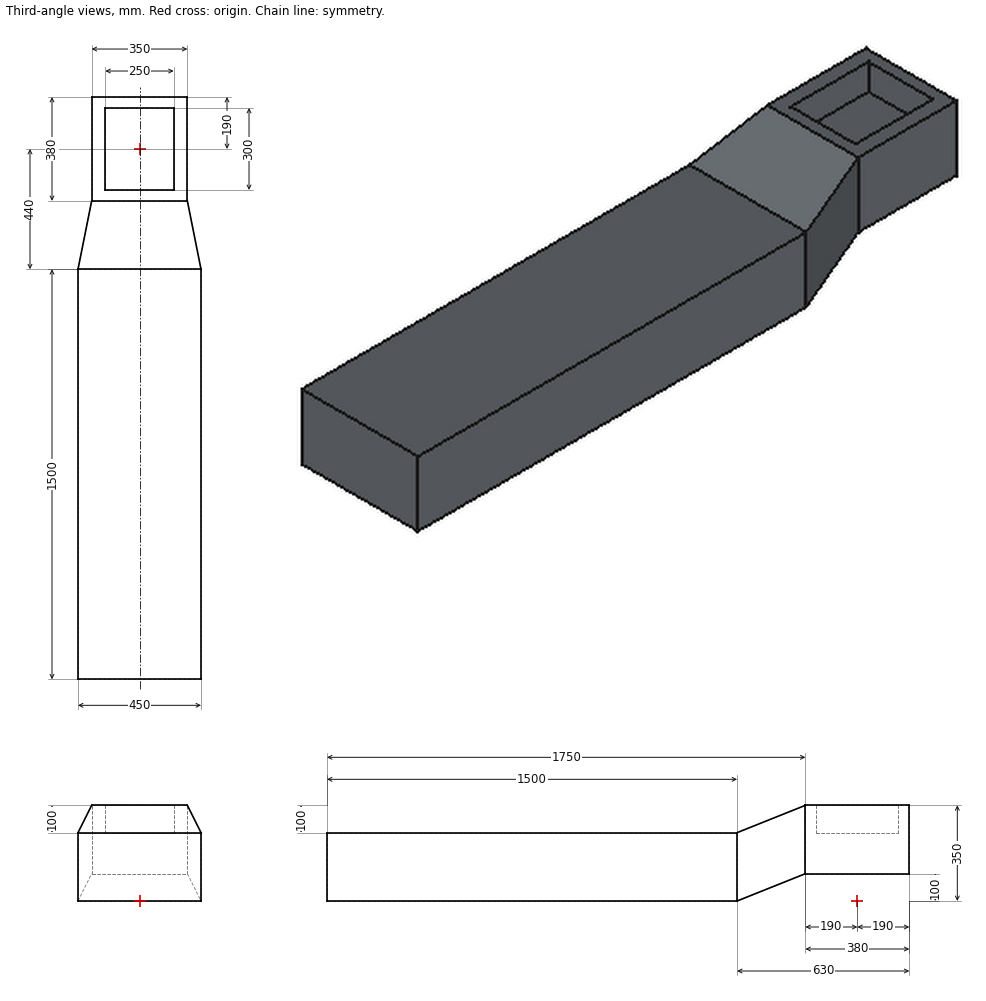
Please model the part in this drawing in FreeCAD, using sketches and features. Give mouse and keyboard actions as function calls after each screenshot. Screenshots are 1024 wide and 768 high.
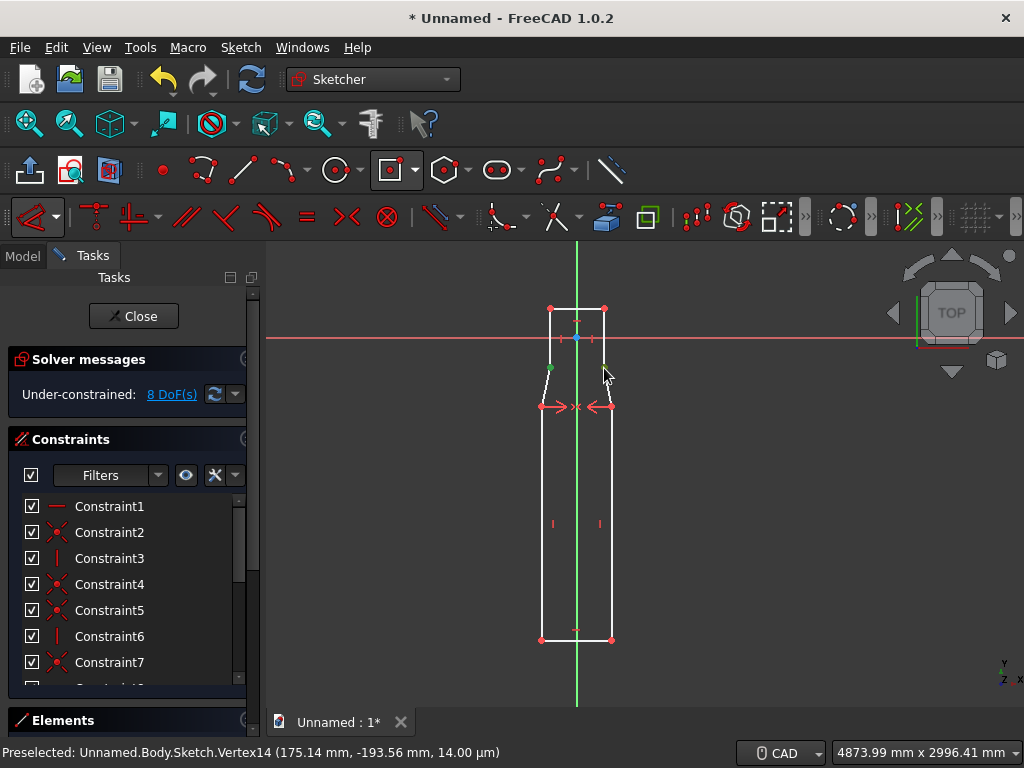
click(577, 591)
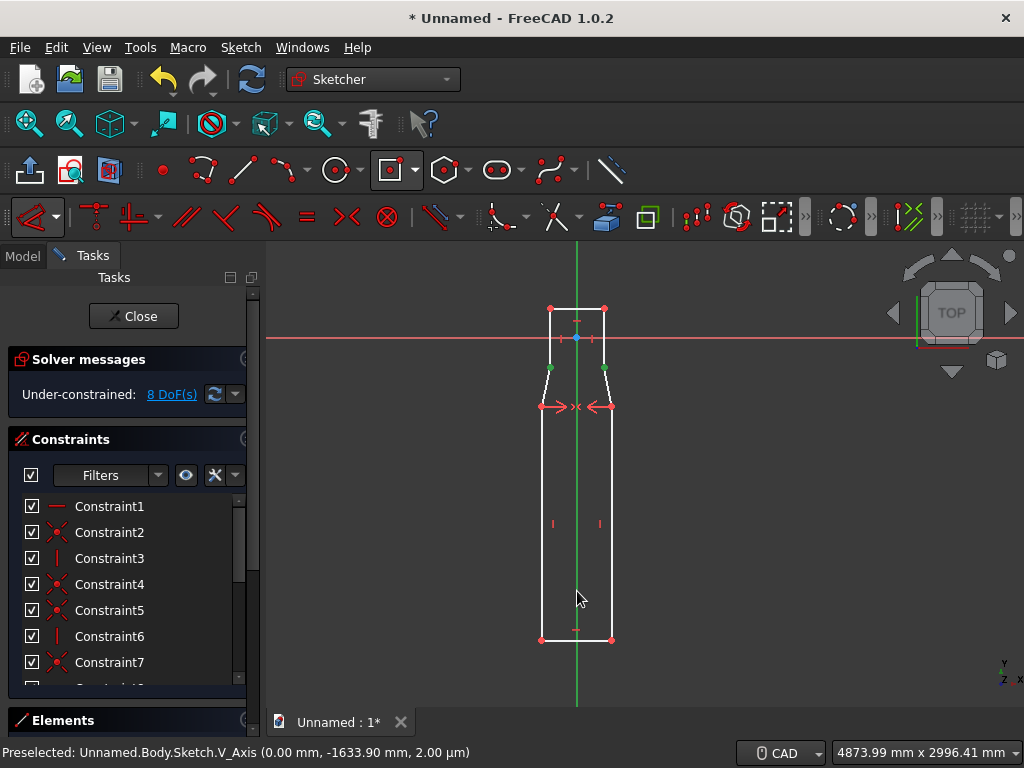
click(348, 218)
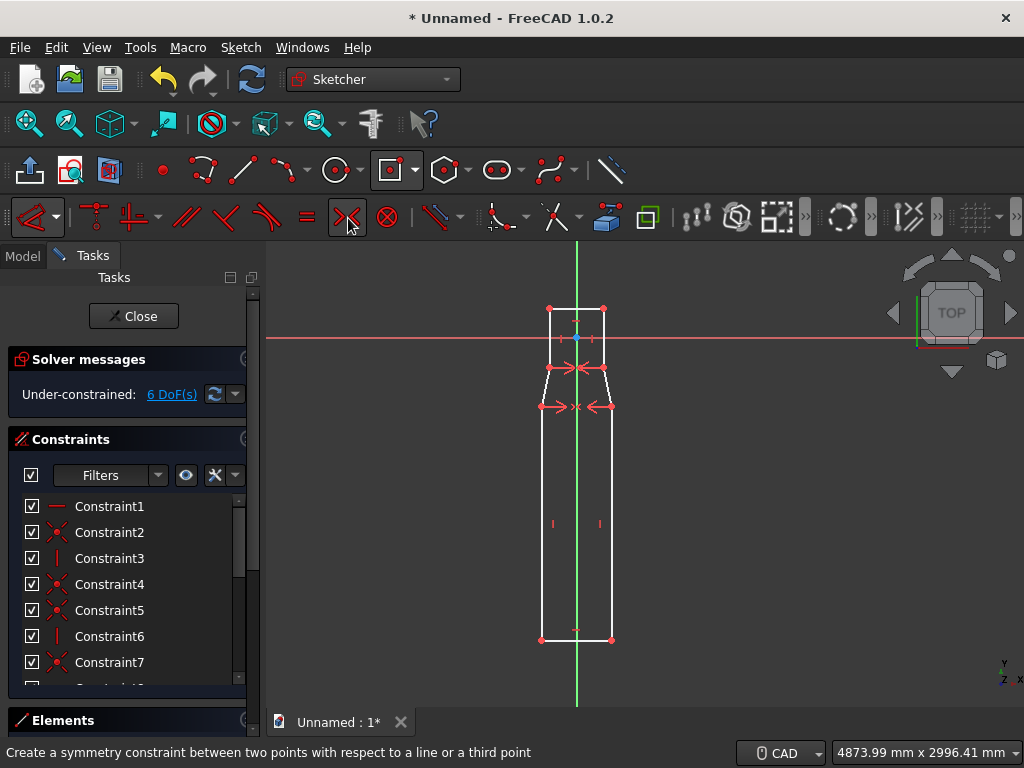
click(32, 218)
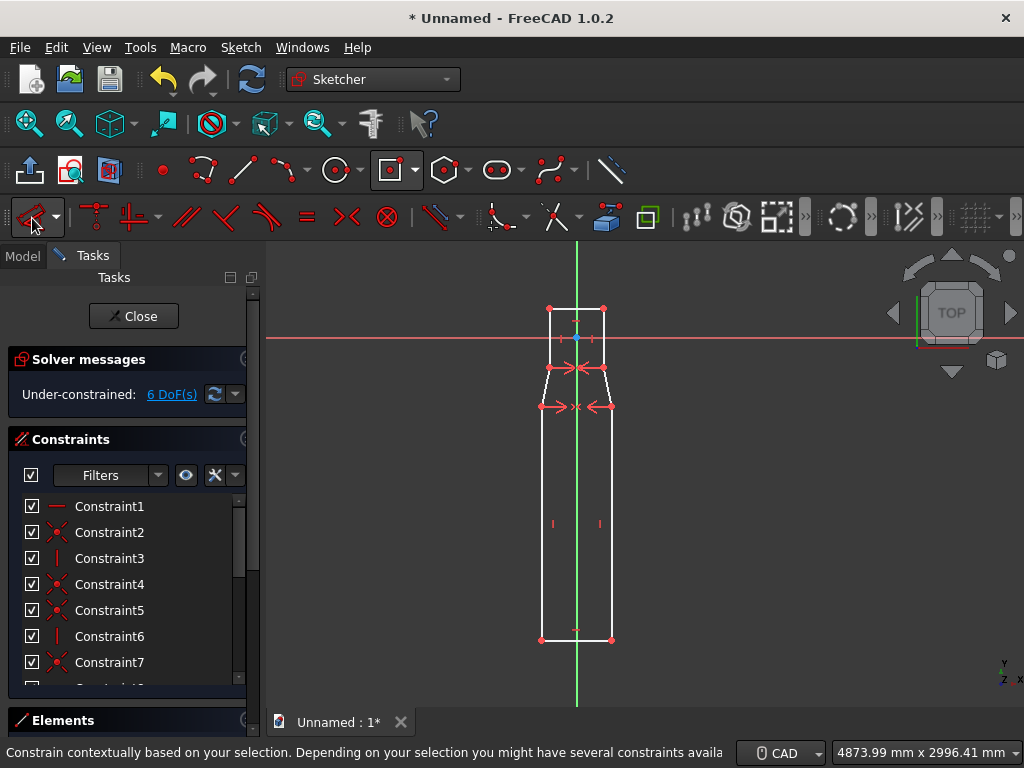
scroll(588, 309, up, 2)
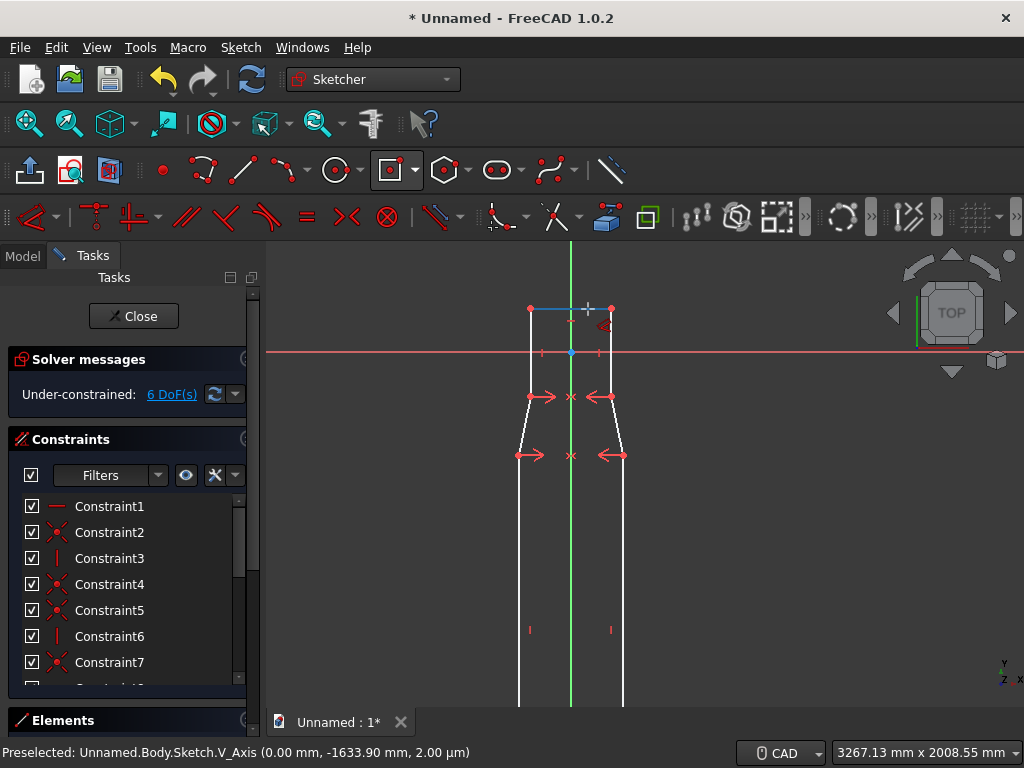
click(587, 309)
click(553, 275)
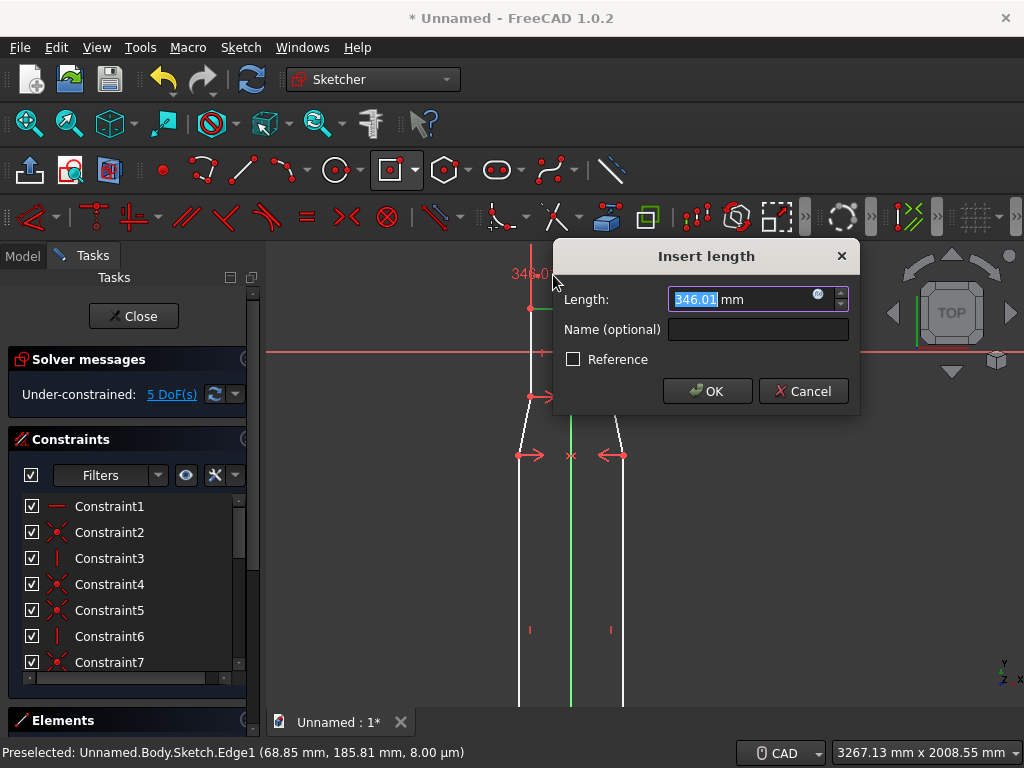
text(350)
key(Return)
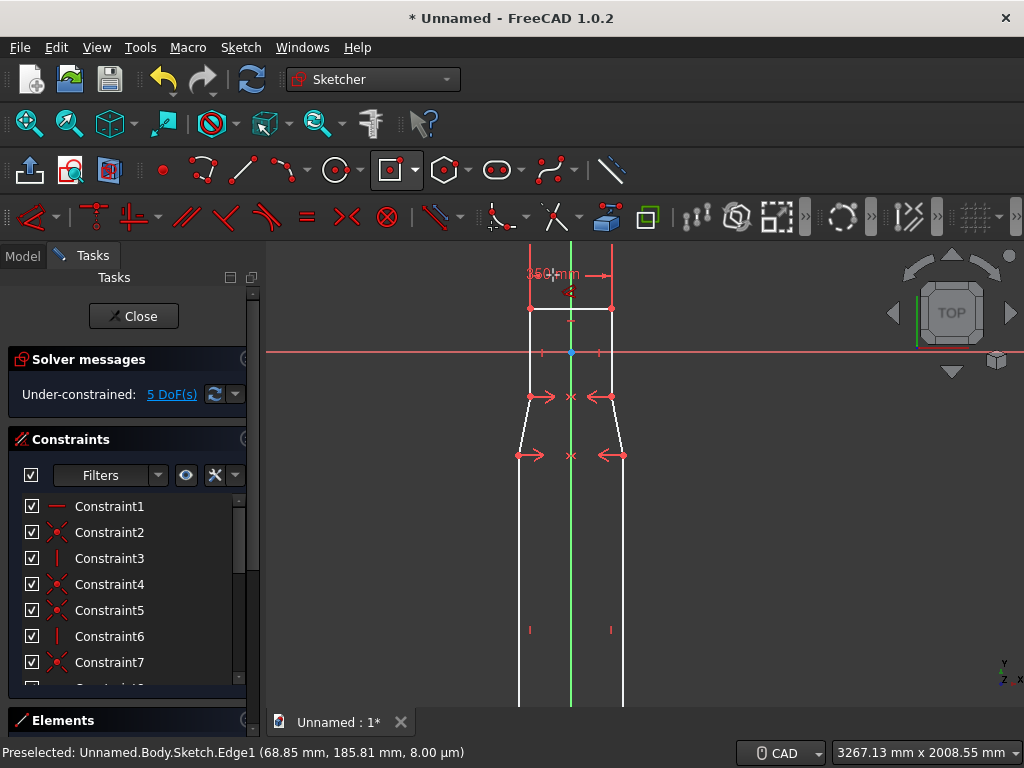
click(530, 335)
click(496, 333)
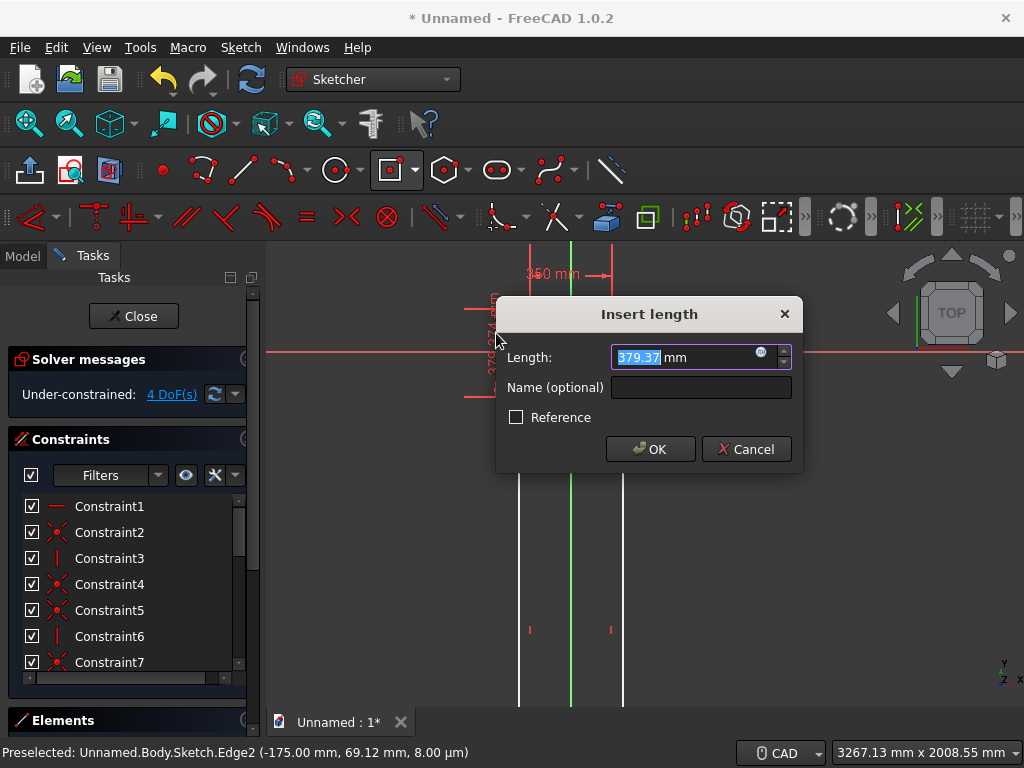
text(380)
key(Return)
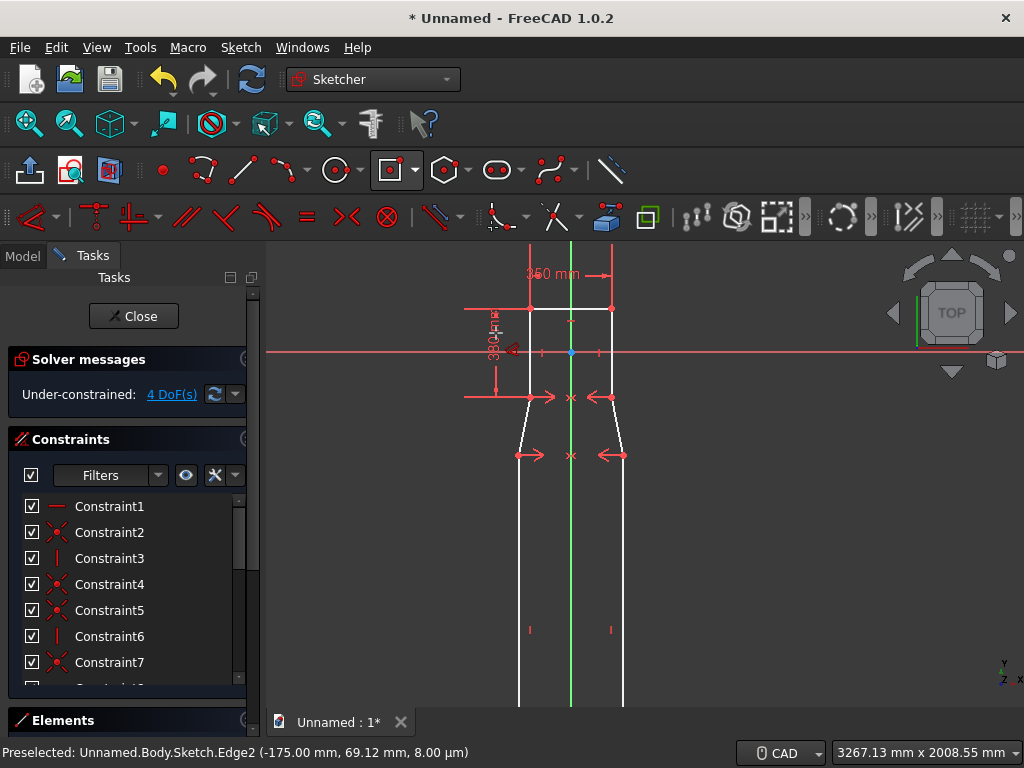
scroll(583, 375, down, 3)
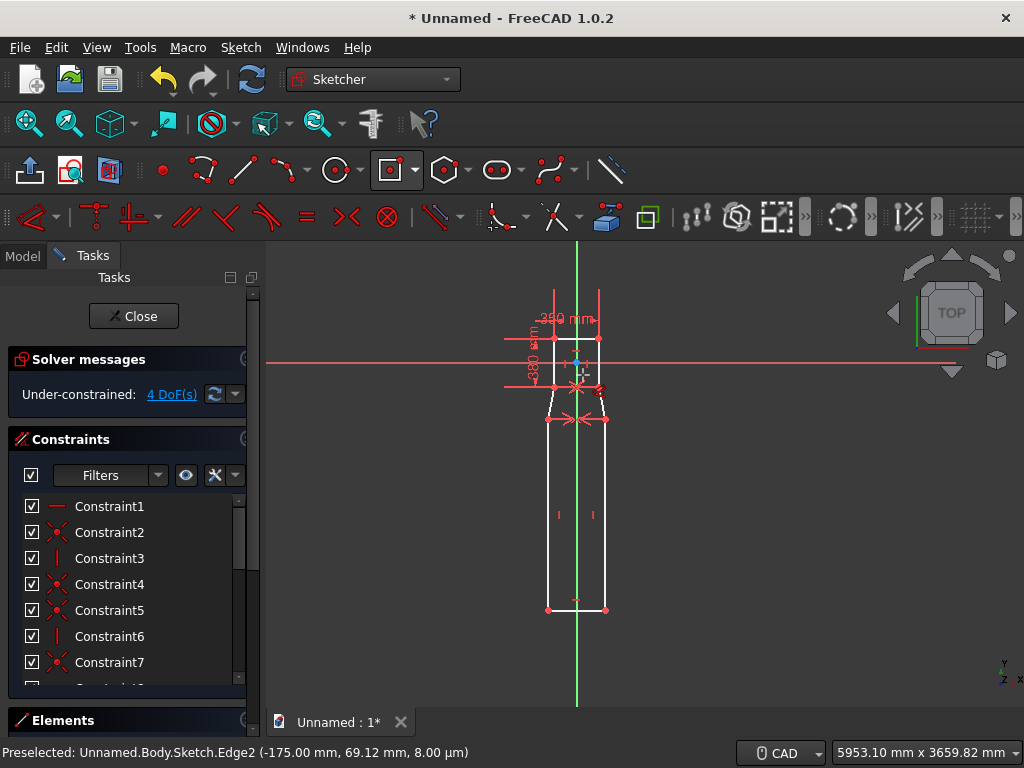
click(565, 611)
click(563, 645)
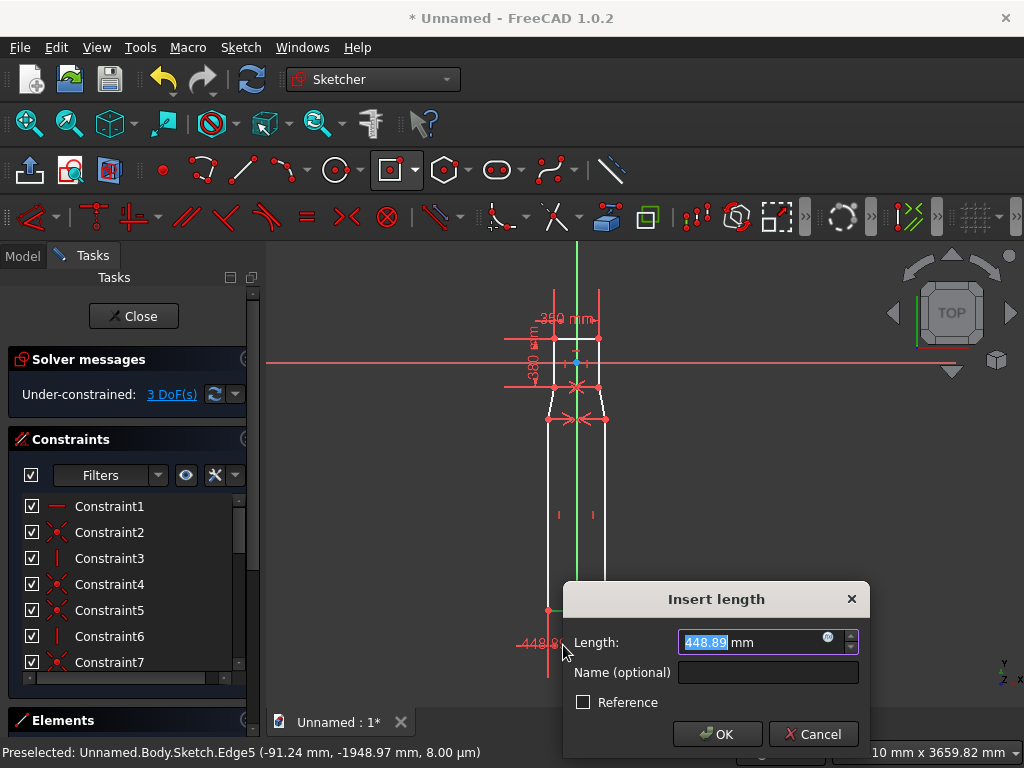
text(450)
key(Return)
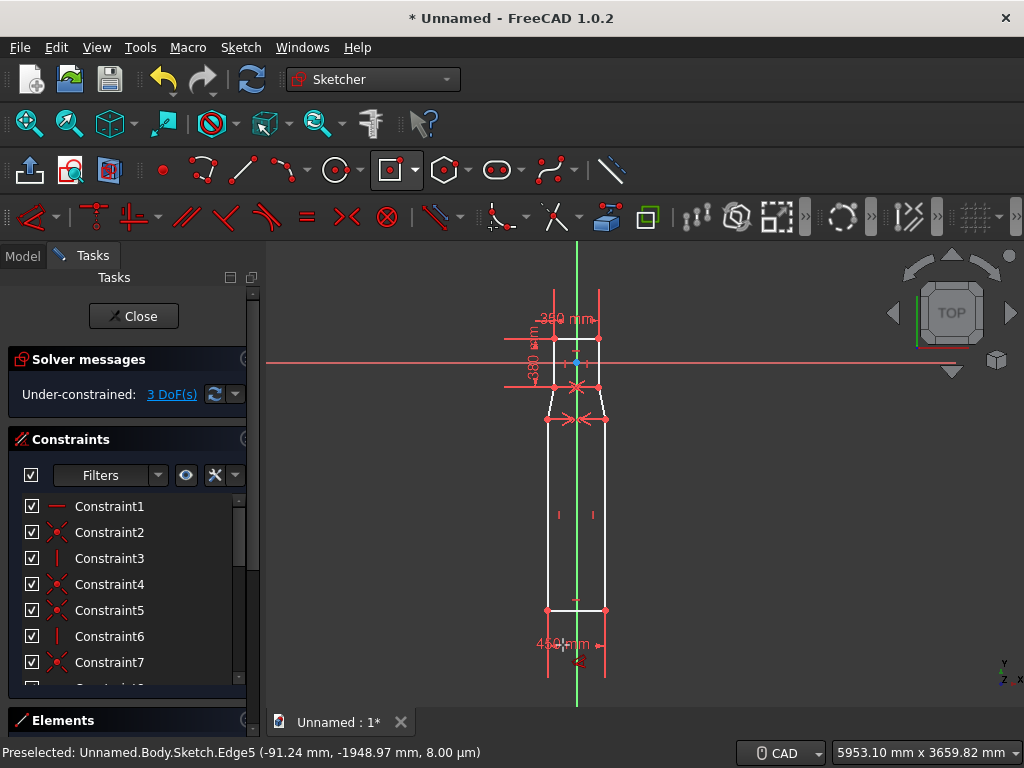
click(548, 477)
click(514, 515)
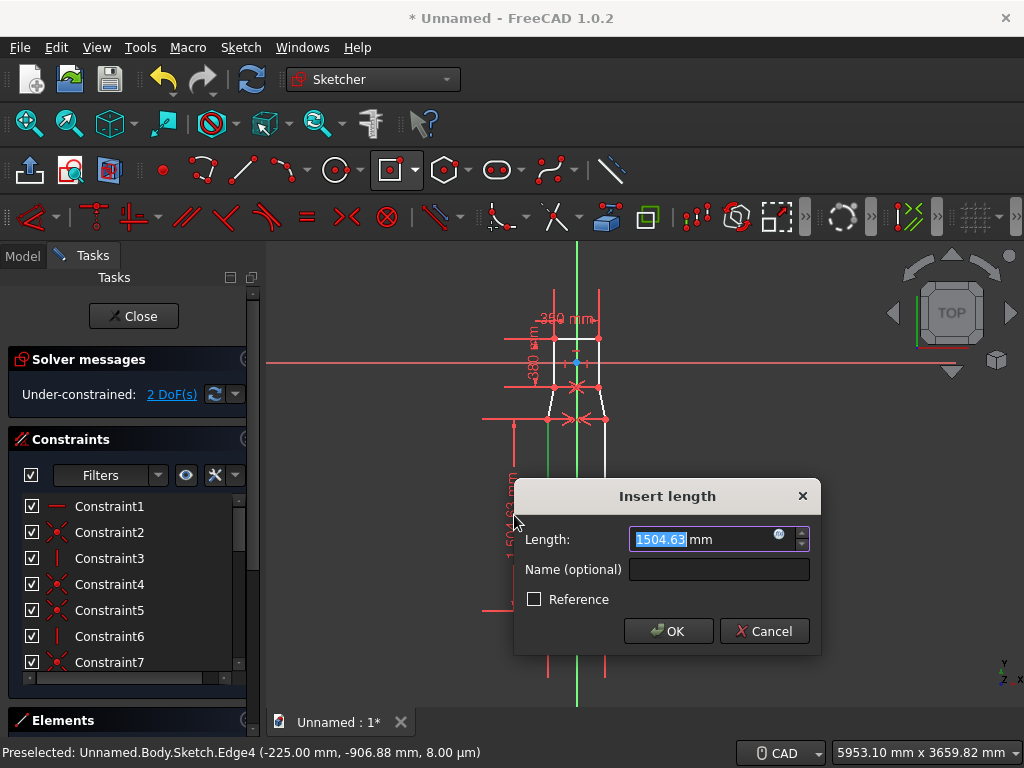
text(1500)
key(Return)